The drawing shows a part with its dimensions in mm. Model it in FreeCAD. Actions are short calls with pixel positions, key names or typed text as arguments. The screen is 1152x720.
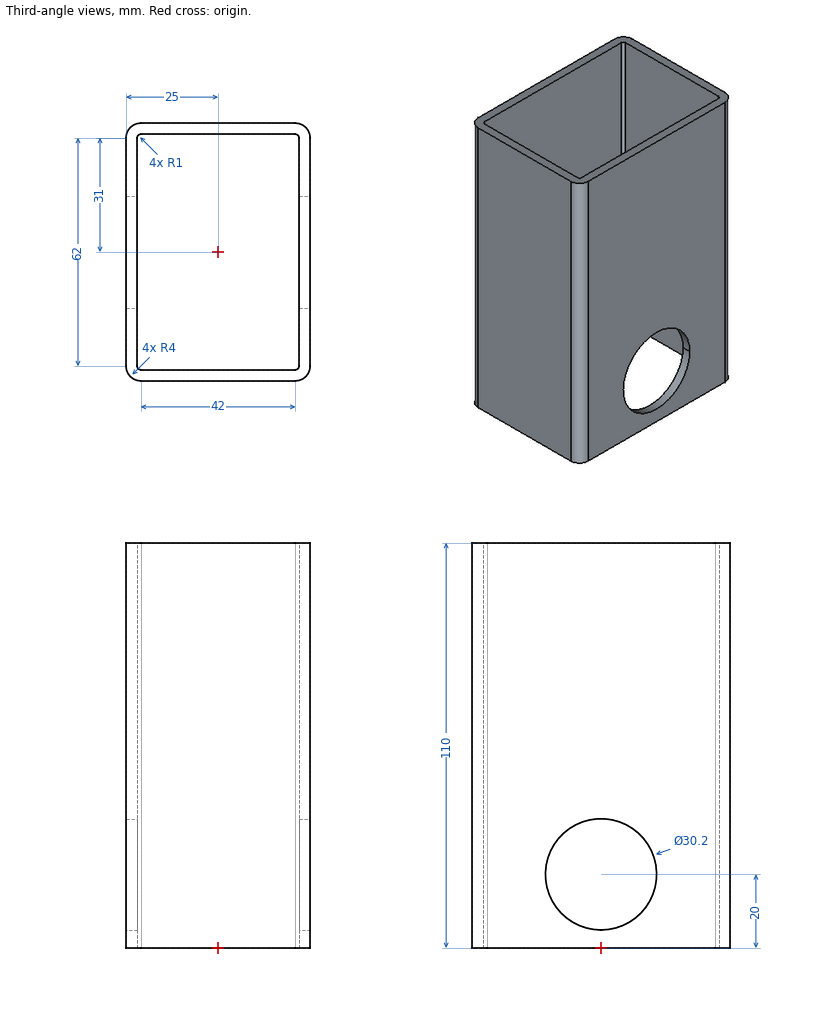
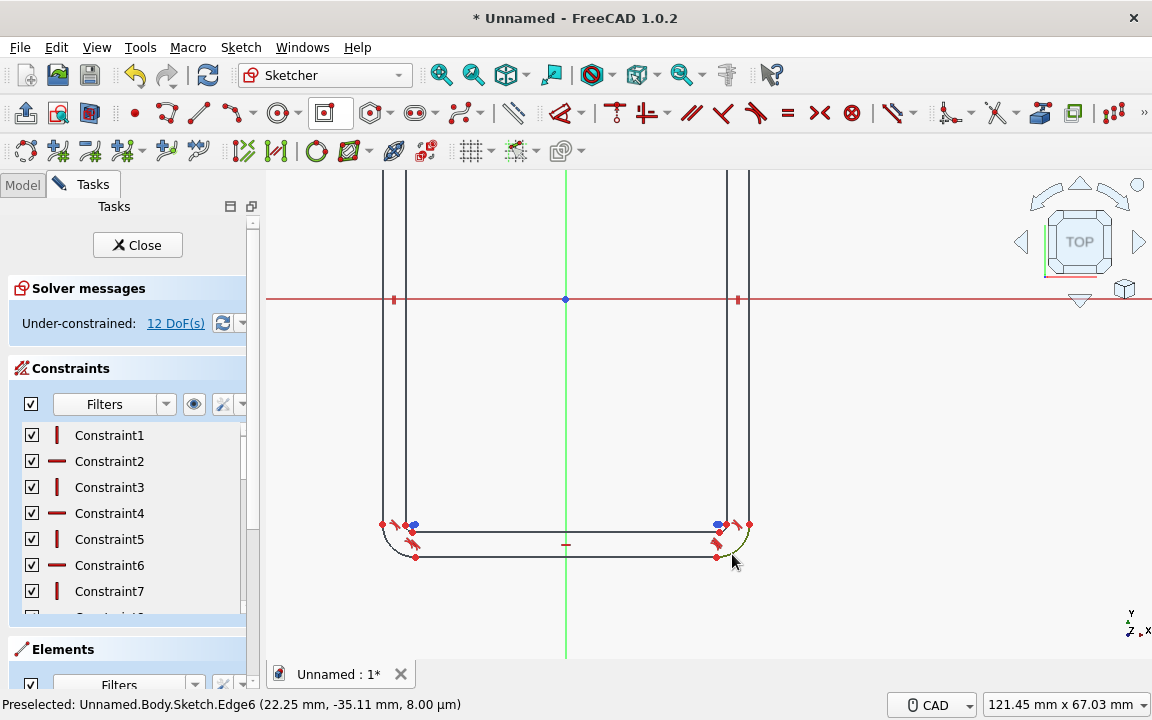
scroll(725, 530, up, 5)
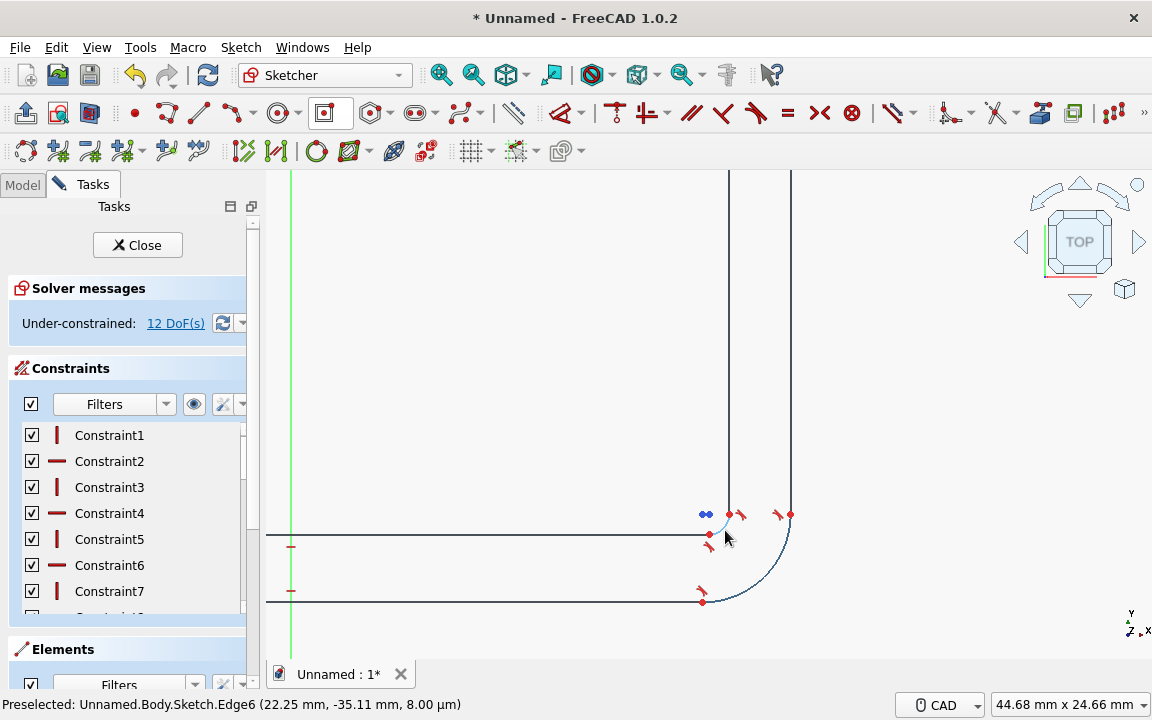
click(723, 529)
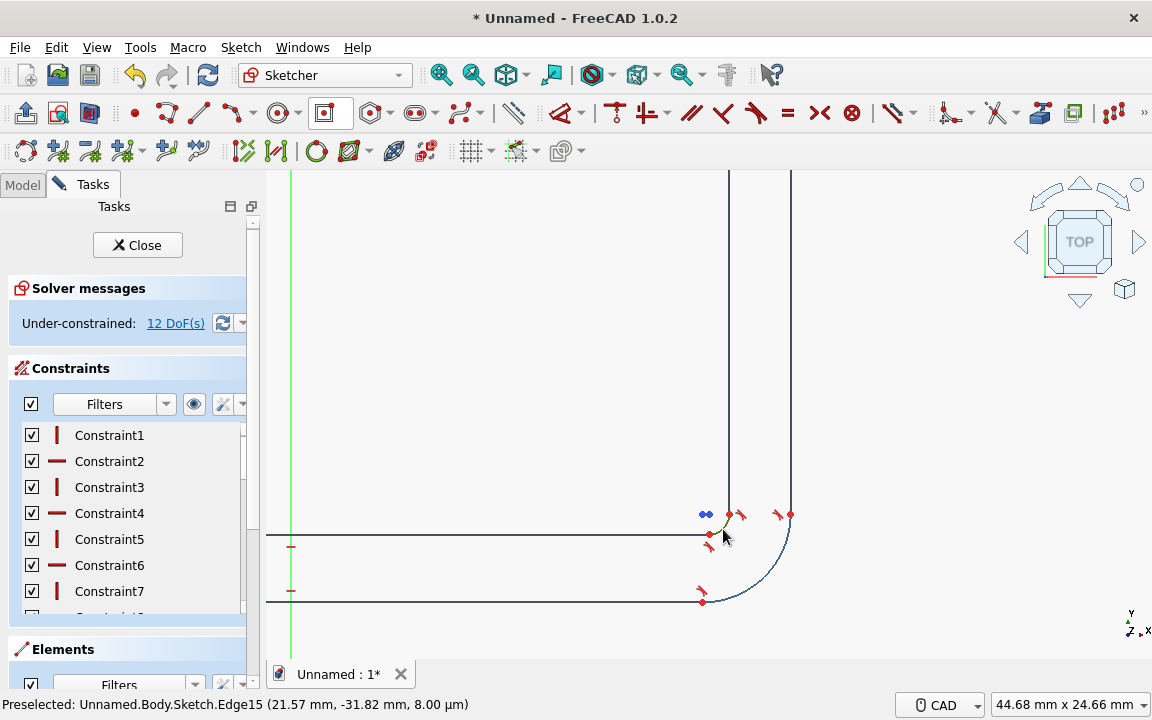
click(616, 114)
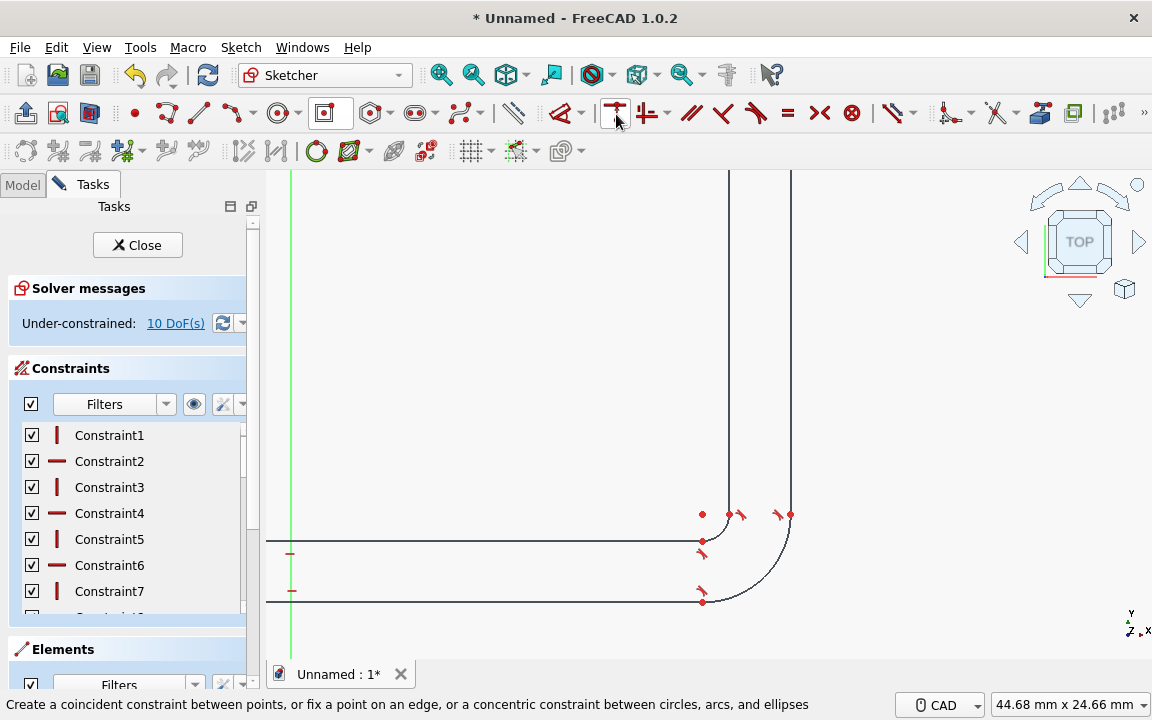
scroll(729, 544, down, 8)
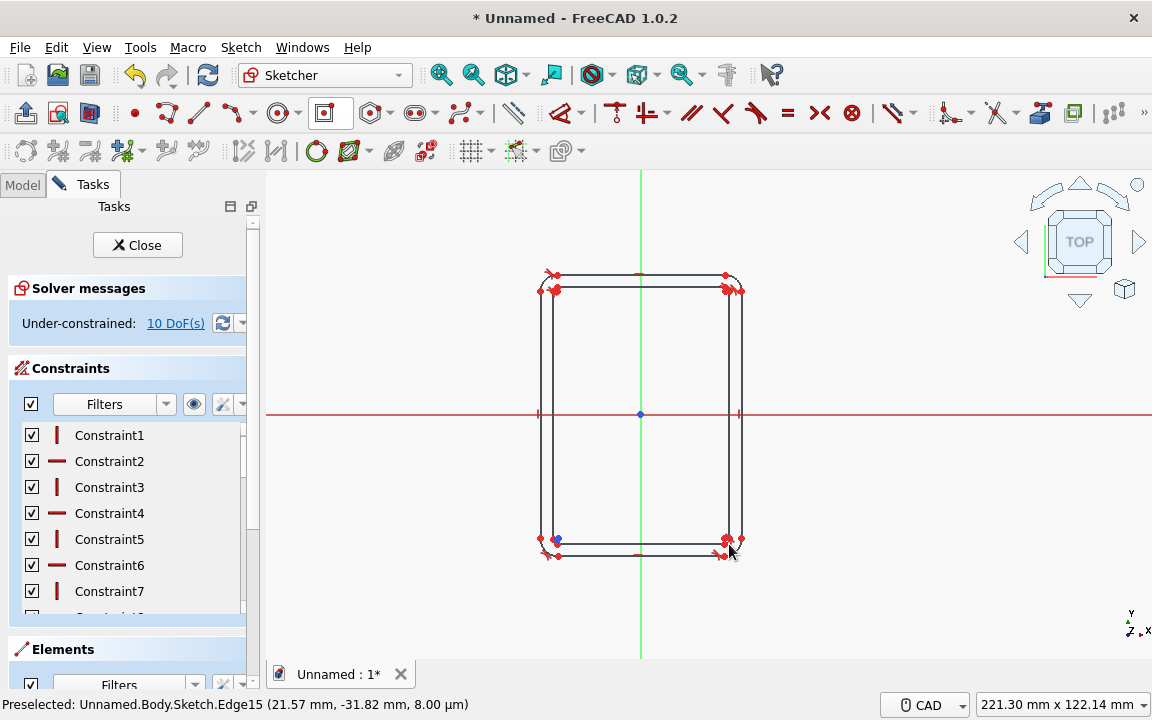
scroll(543, 547, up, 3)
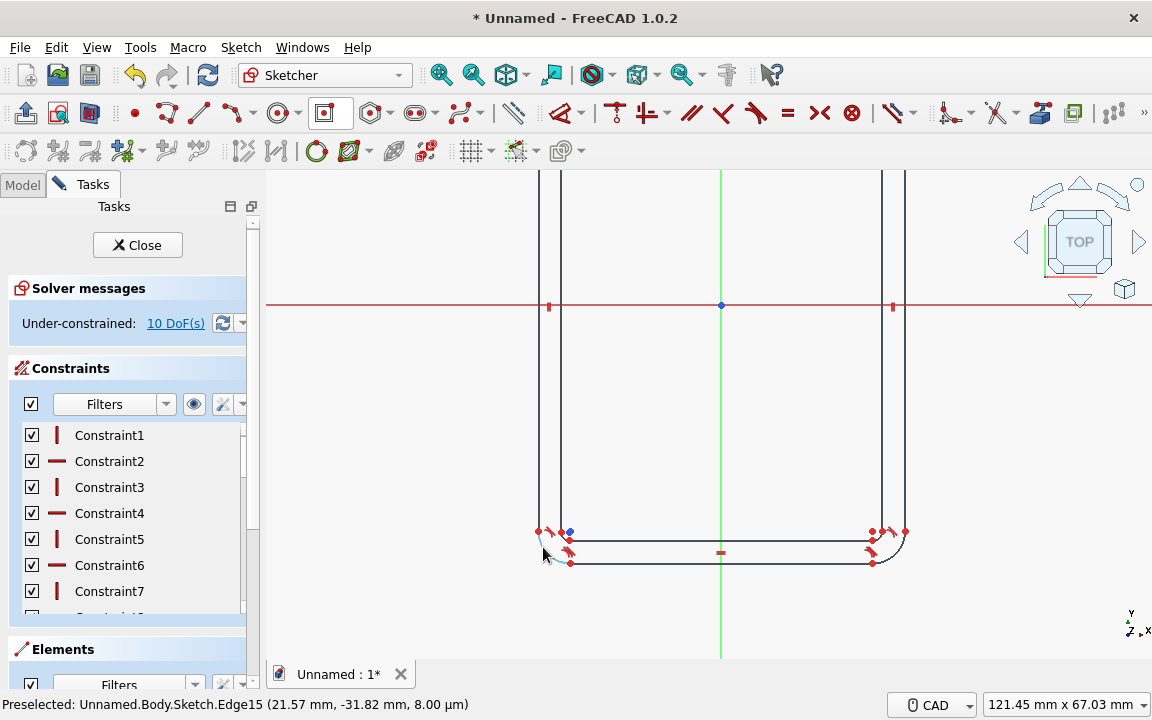
click(542, 546)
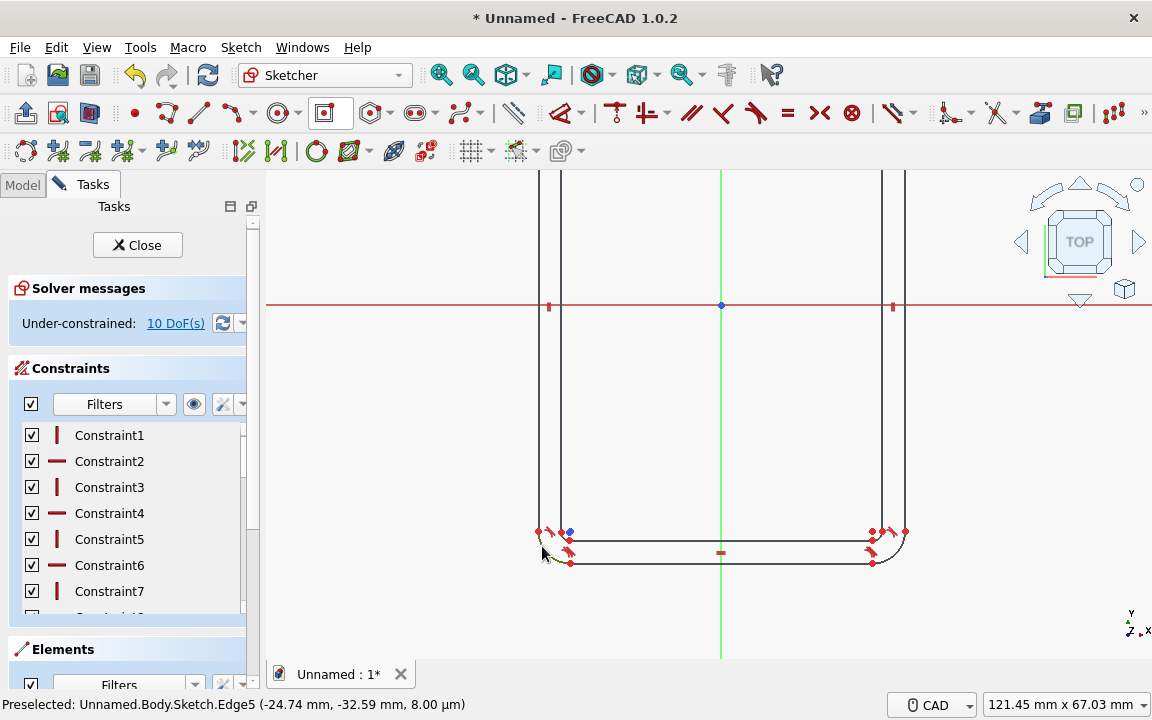
click(887, 560)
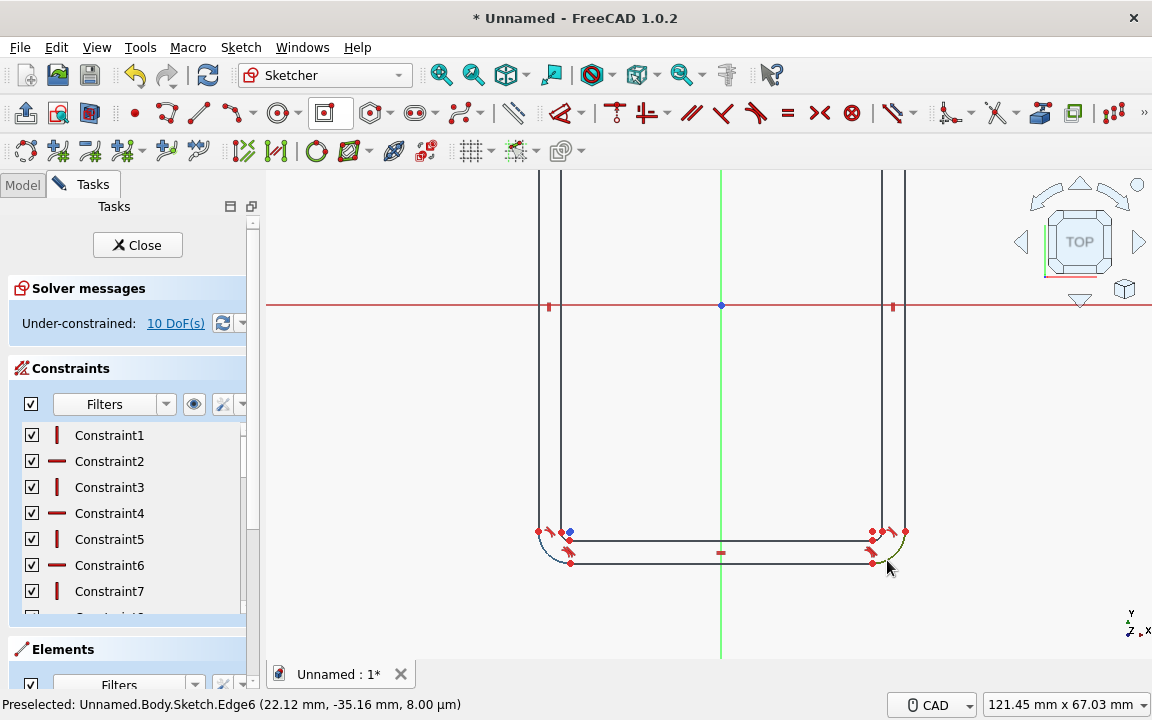
scroll(542, 547, down, 3)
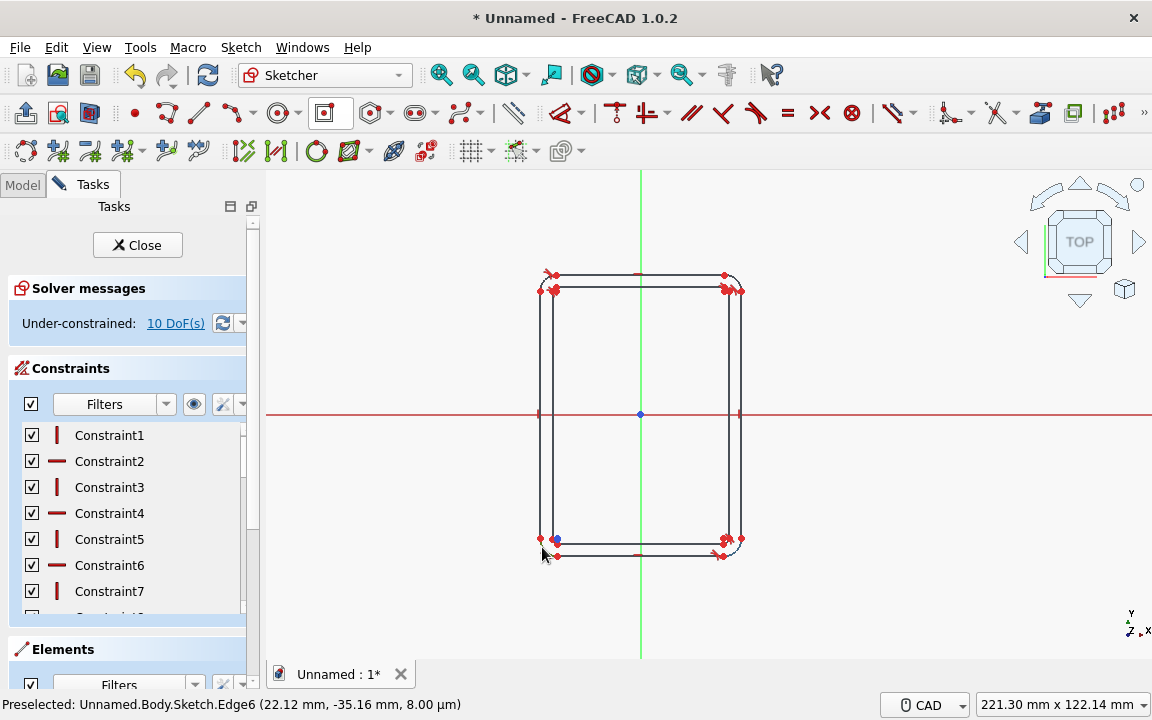
scroll(740, 284, up, 3)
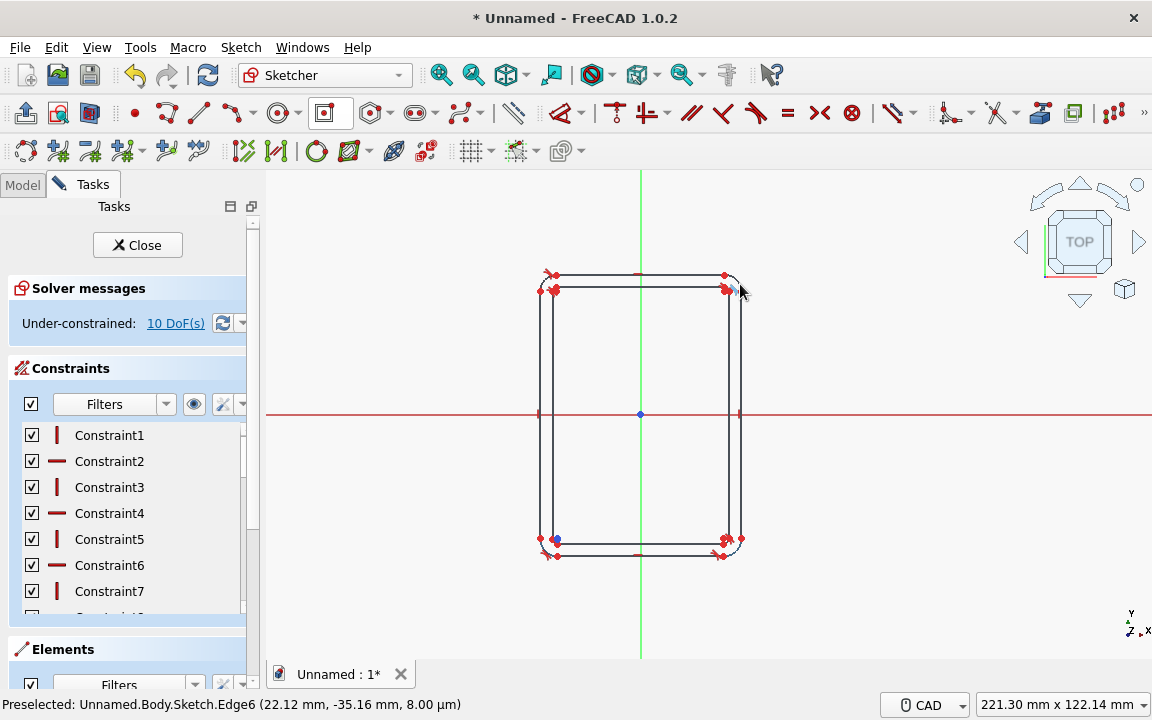
click(739, 284)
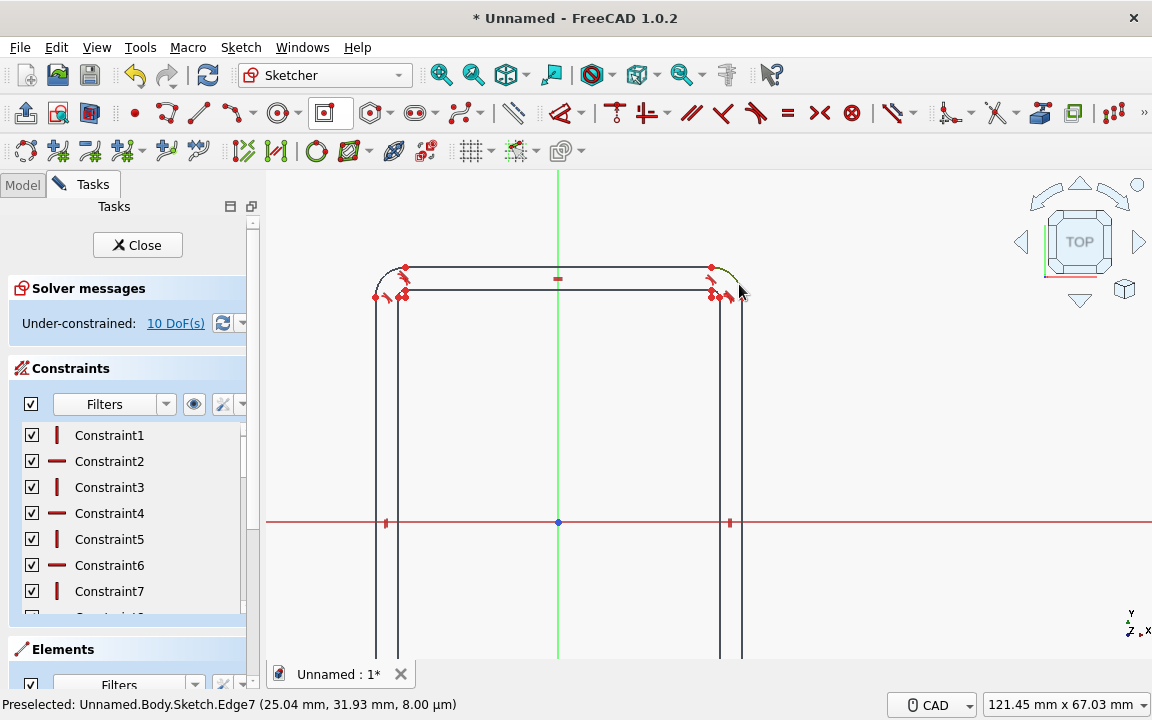
click(392, 271)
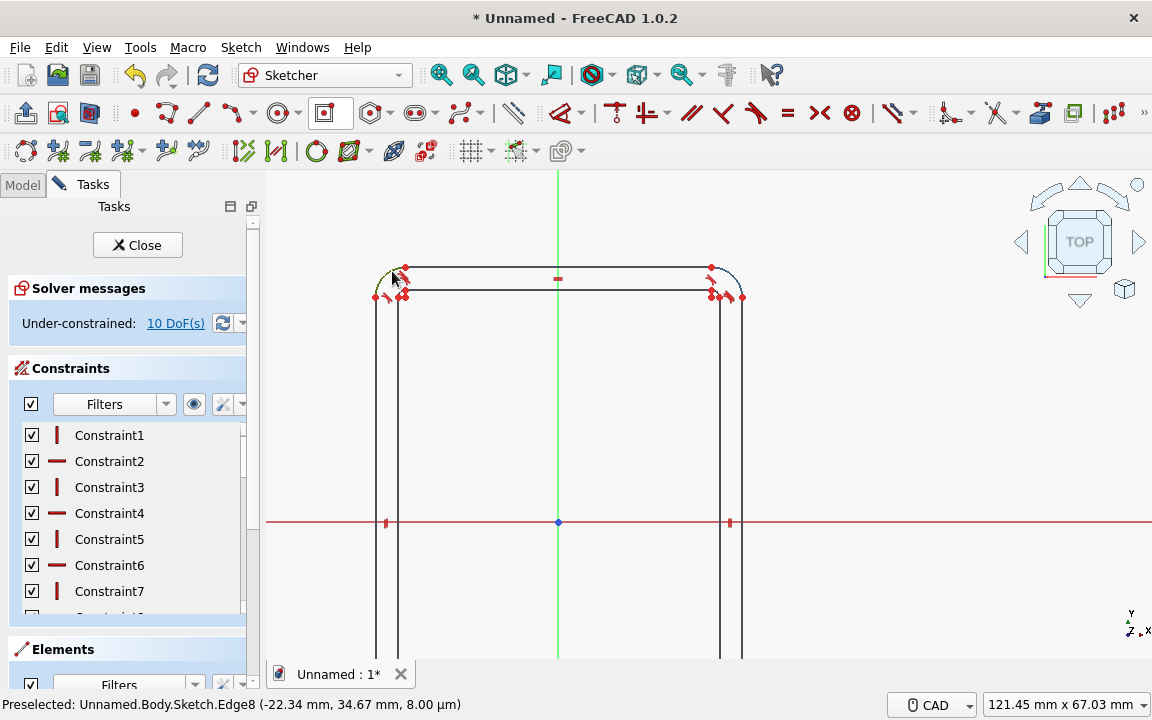
key(e)